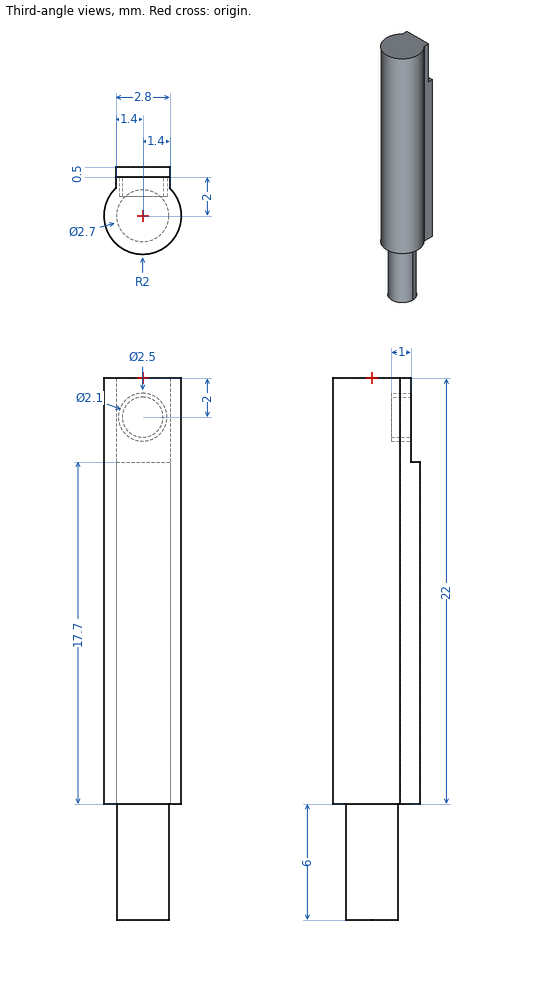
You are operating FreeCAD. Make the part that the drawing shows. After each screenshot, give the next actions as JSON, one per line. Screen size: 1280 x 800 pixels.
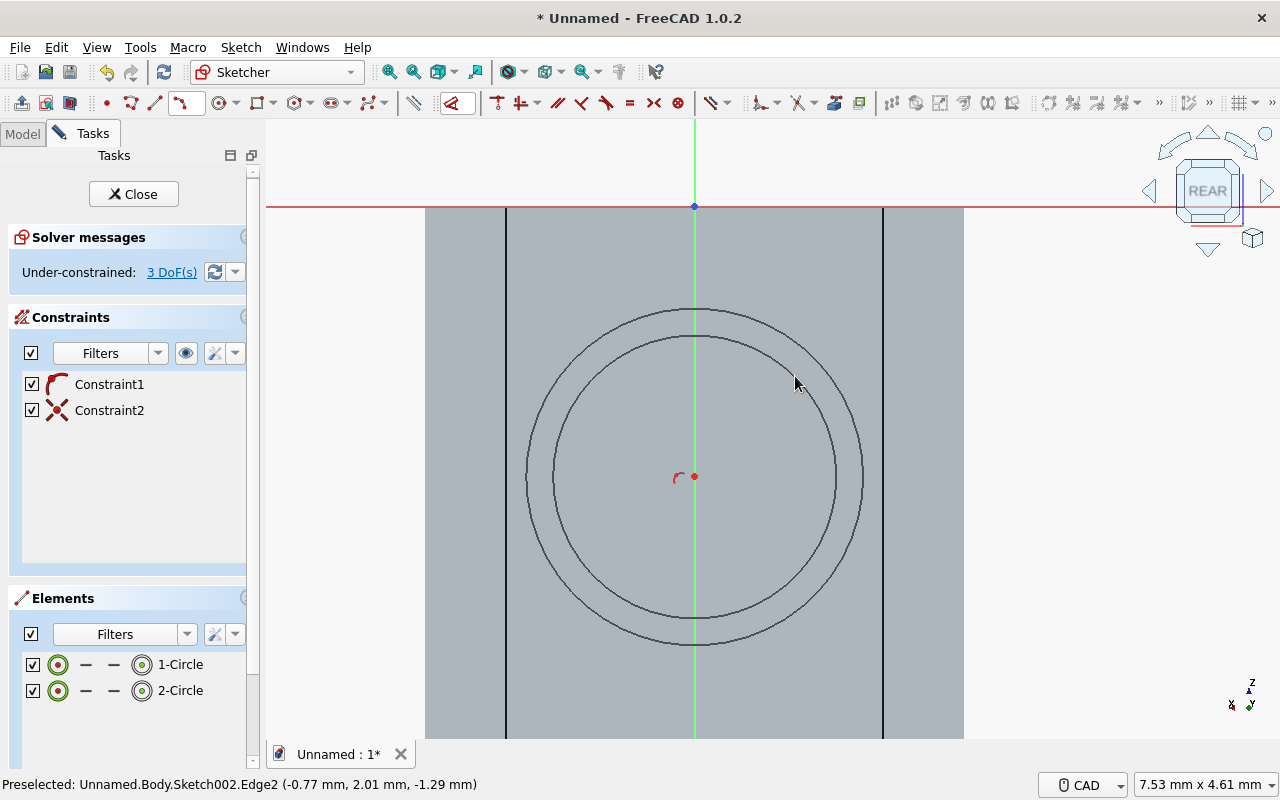
{"action": "left_click", "coordinate": [813, 357]}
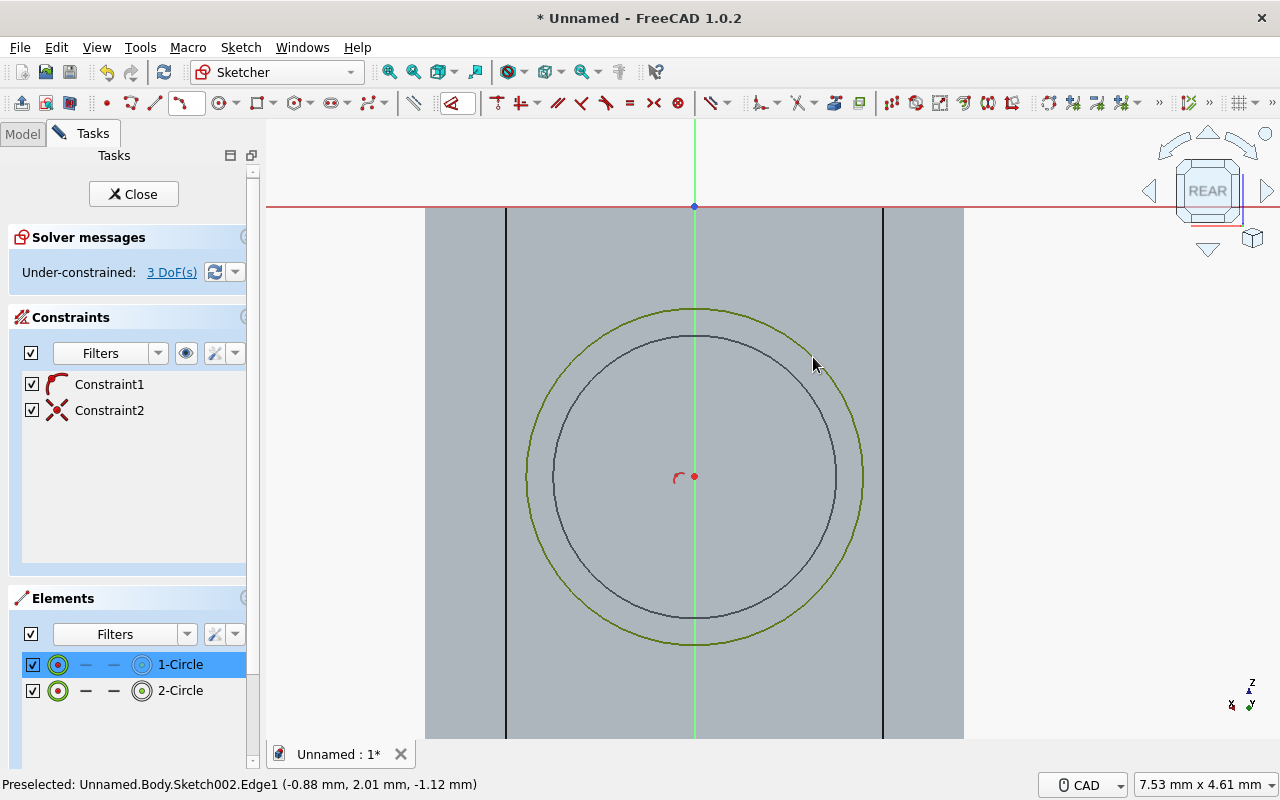
{"action": "key", "text": "k o"}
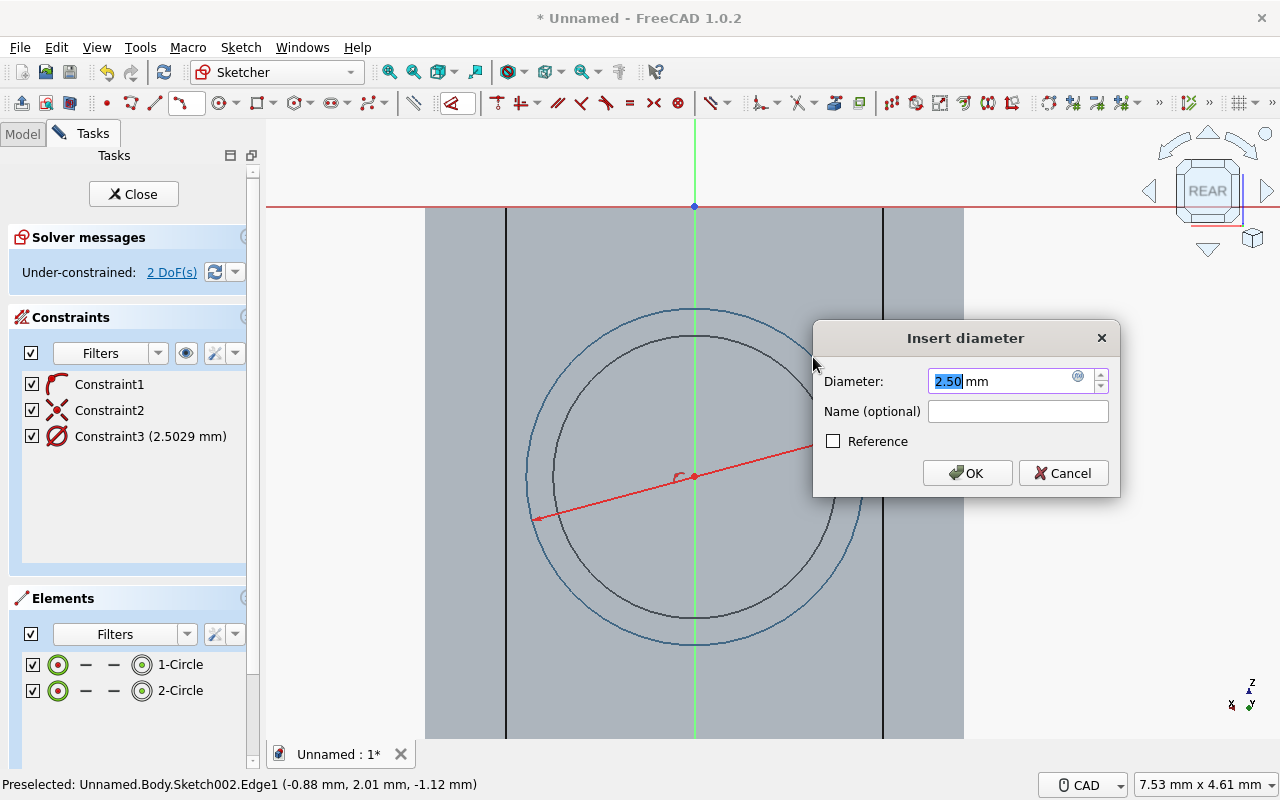
{"action": "type", "text": "2.5"}
{"action": "key", "text": "Return"}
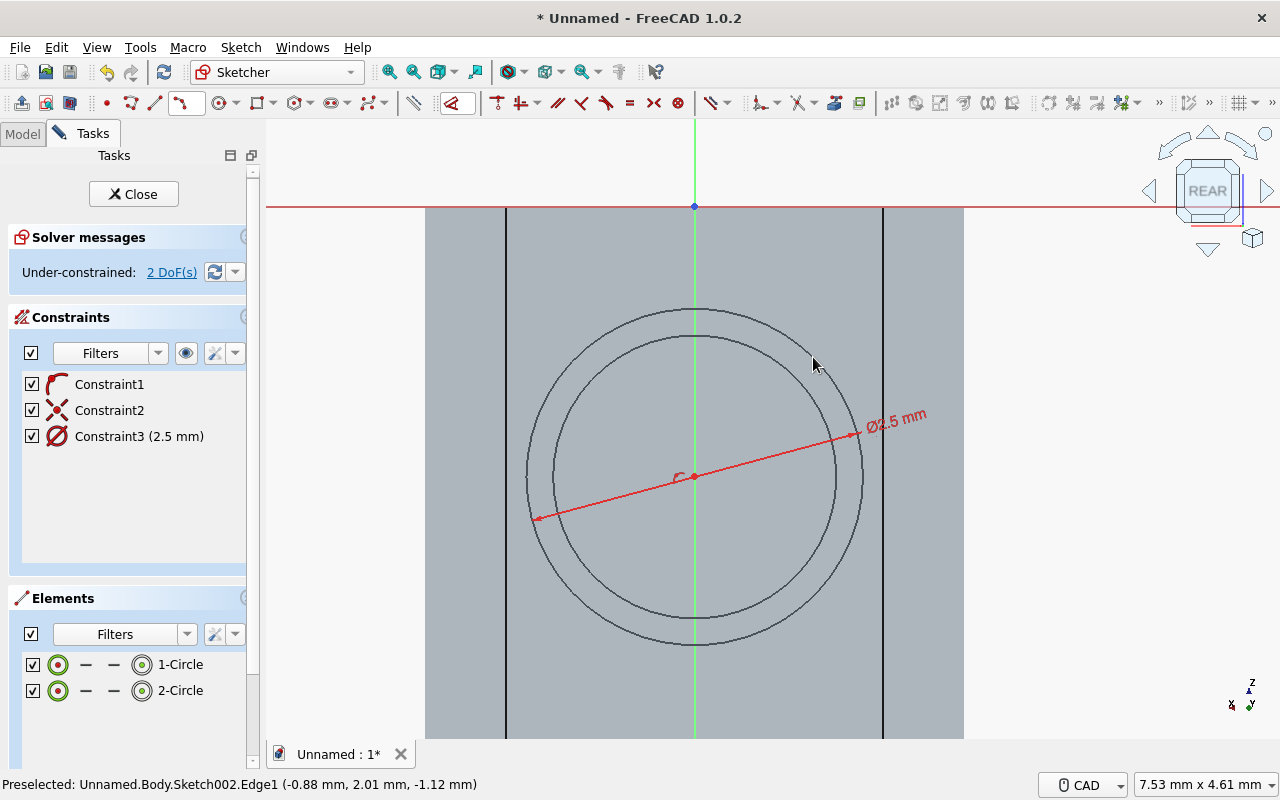
{"action": "left_click", "coordinate": [795, 377]}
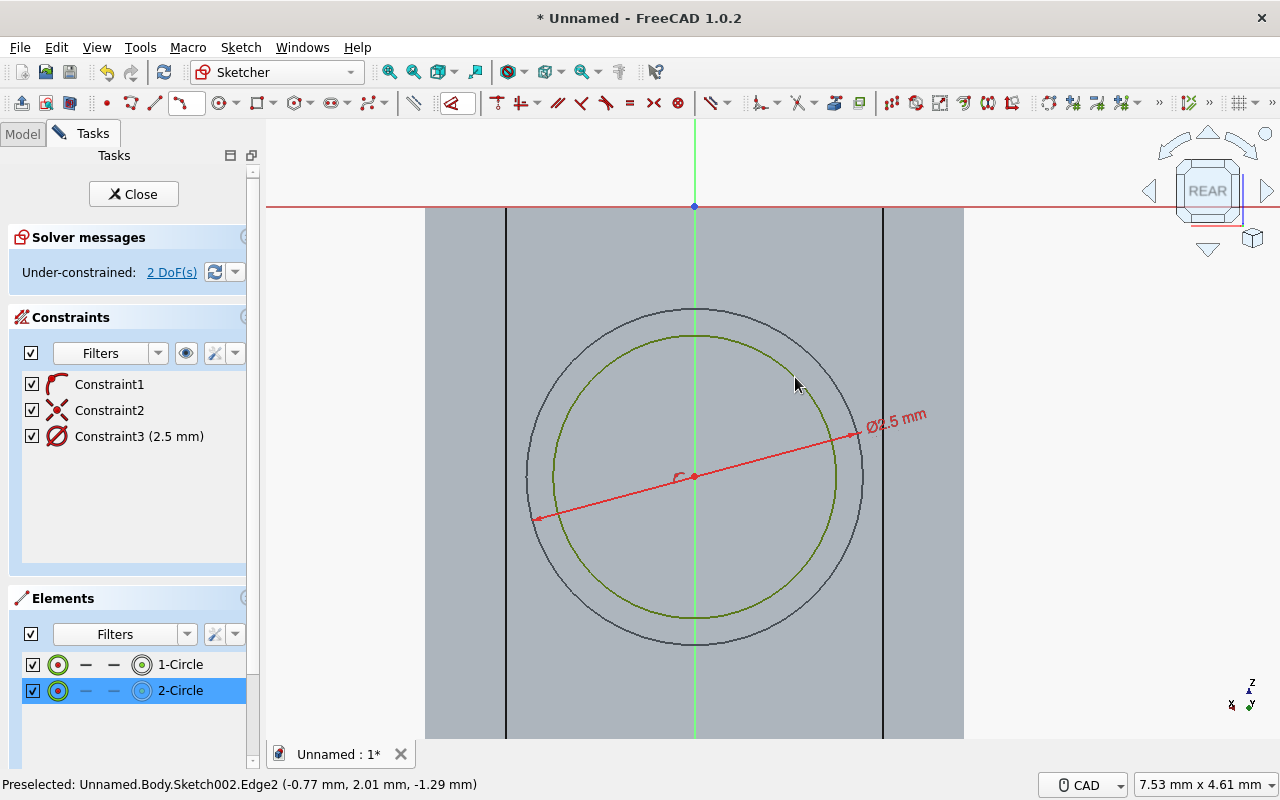
{"action": "left_click", "coordinate": [470, 104]}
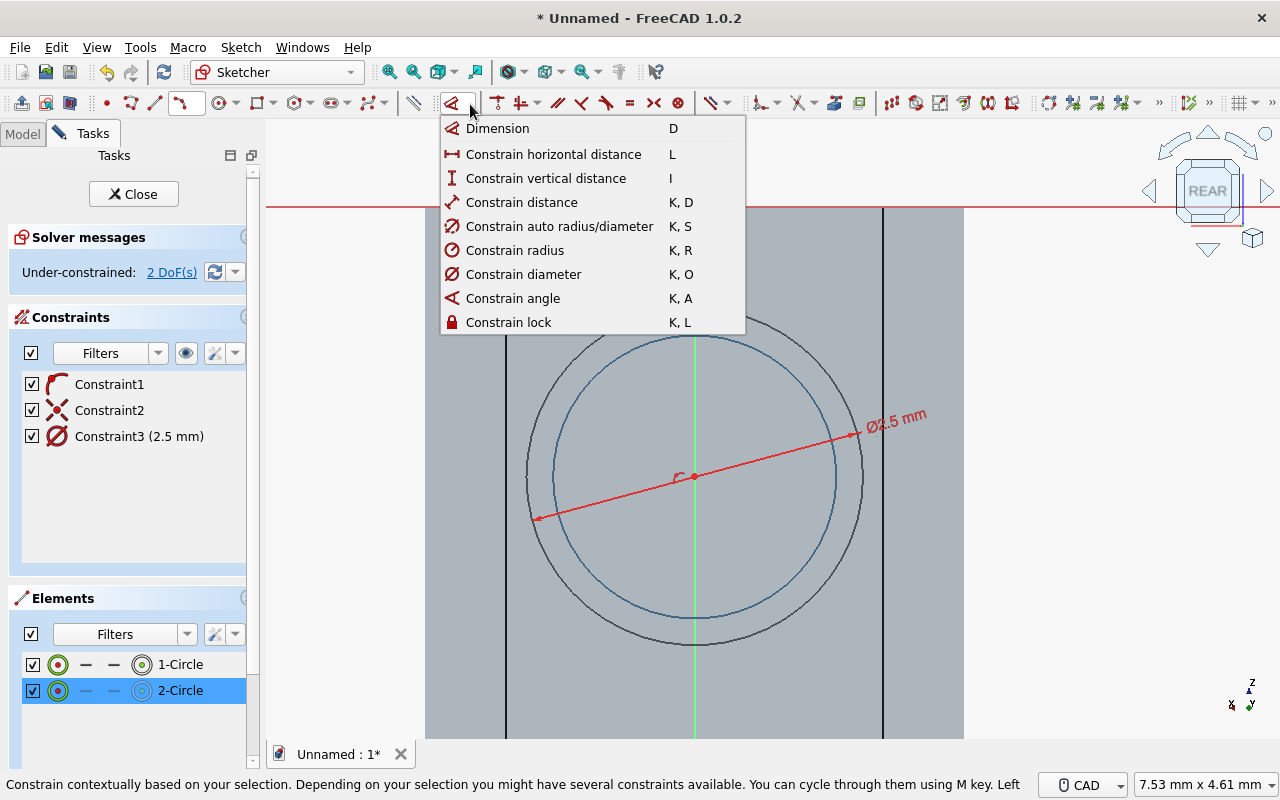
{"action": "left_click", "coordinate": [593, 274]}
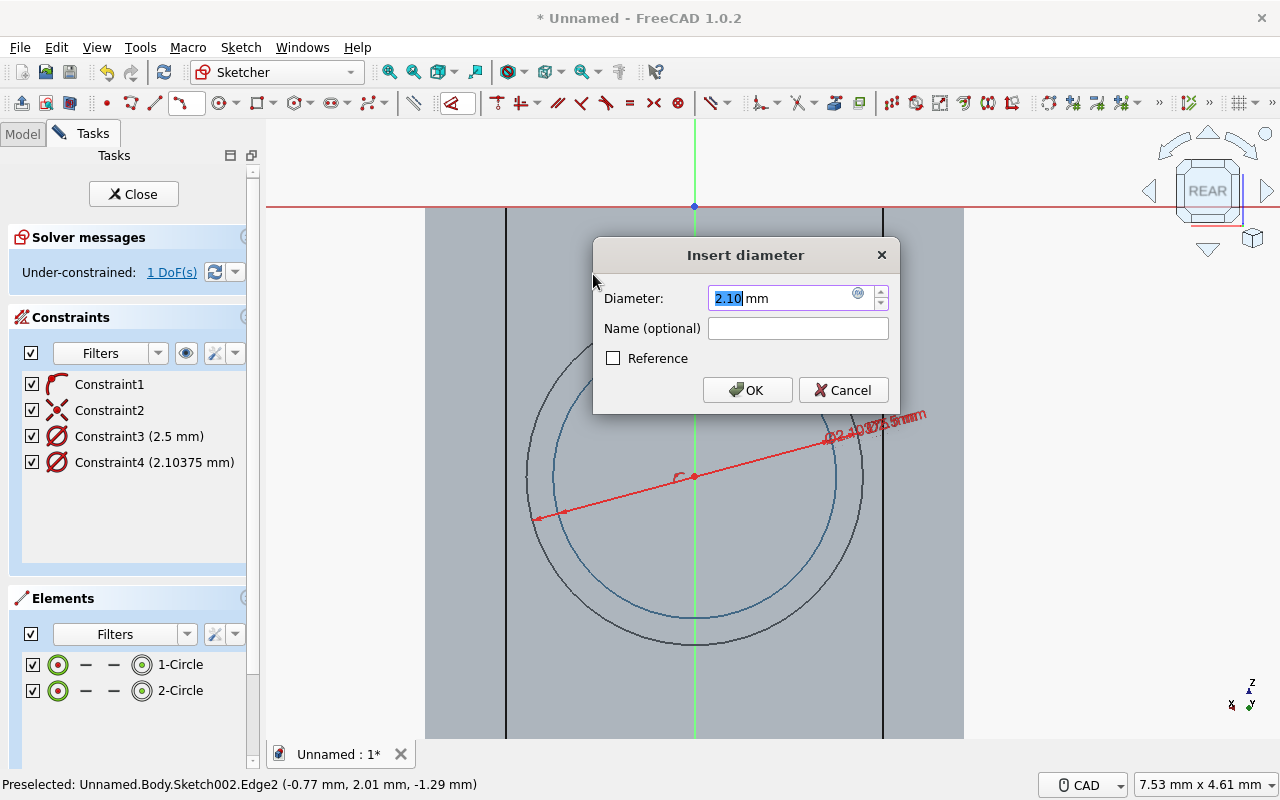
{"action": "type", "text": "2.1"}
{"action": "key", "text": "Return"}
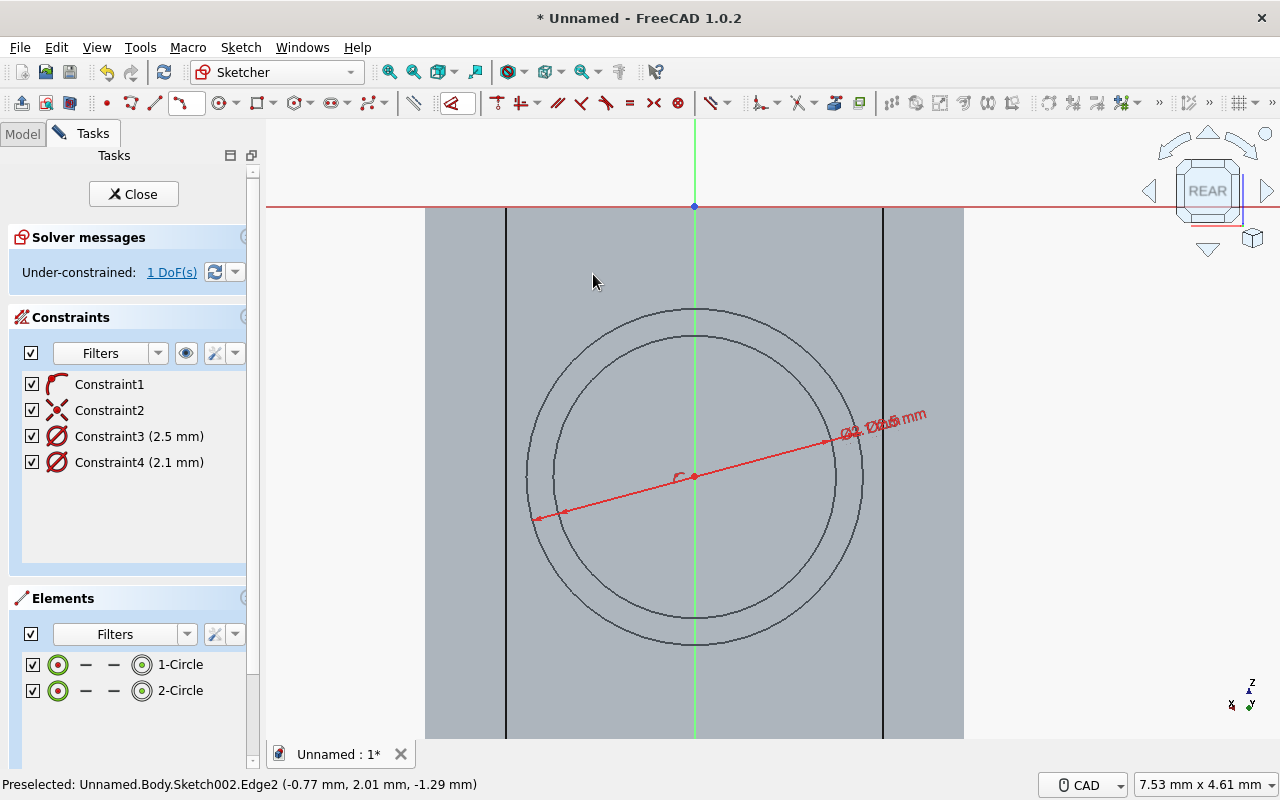
{"action": "left_click", "coordinate": [695, 477]}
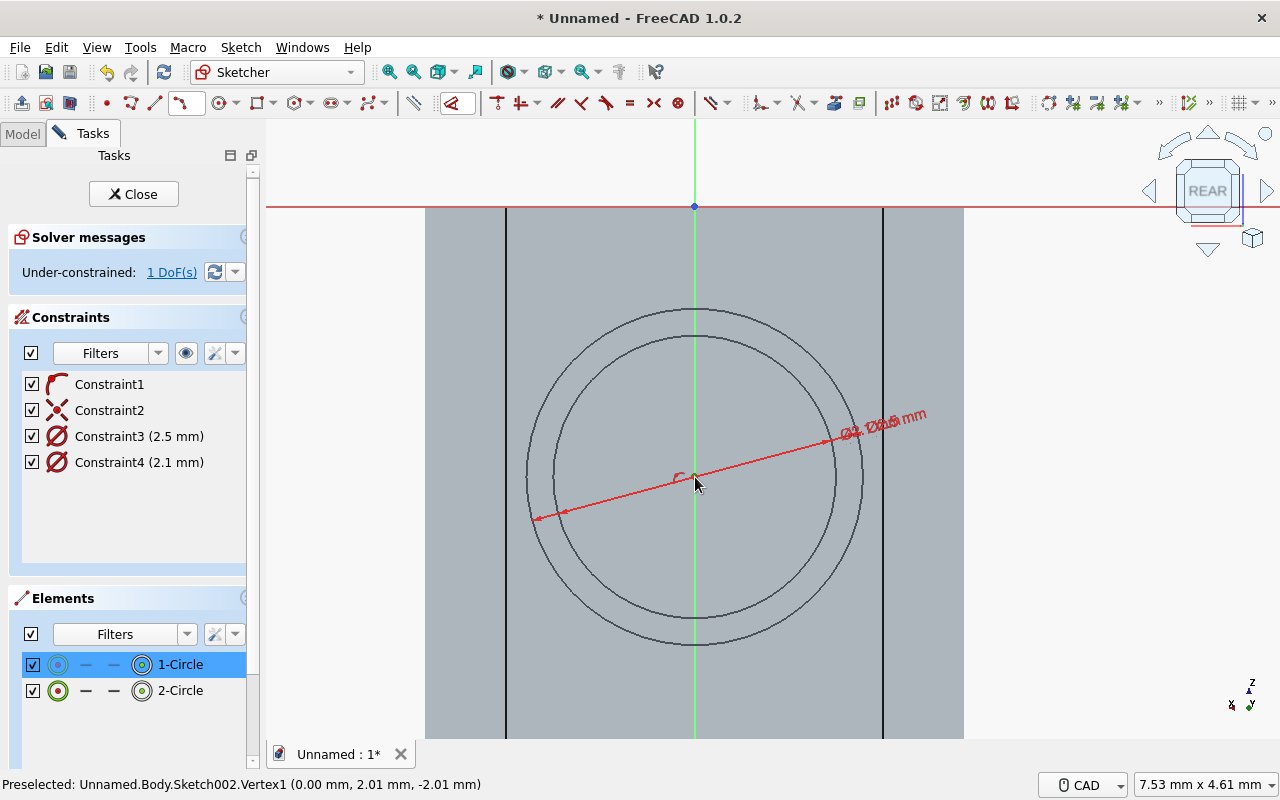
{"action": "left_click", "coordinate": [470, 104]}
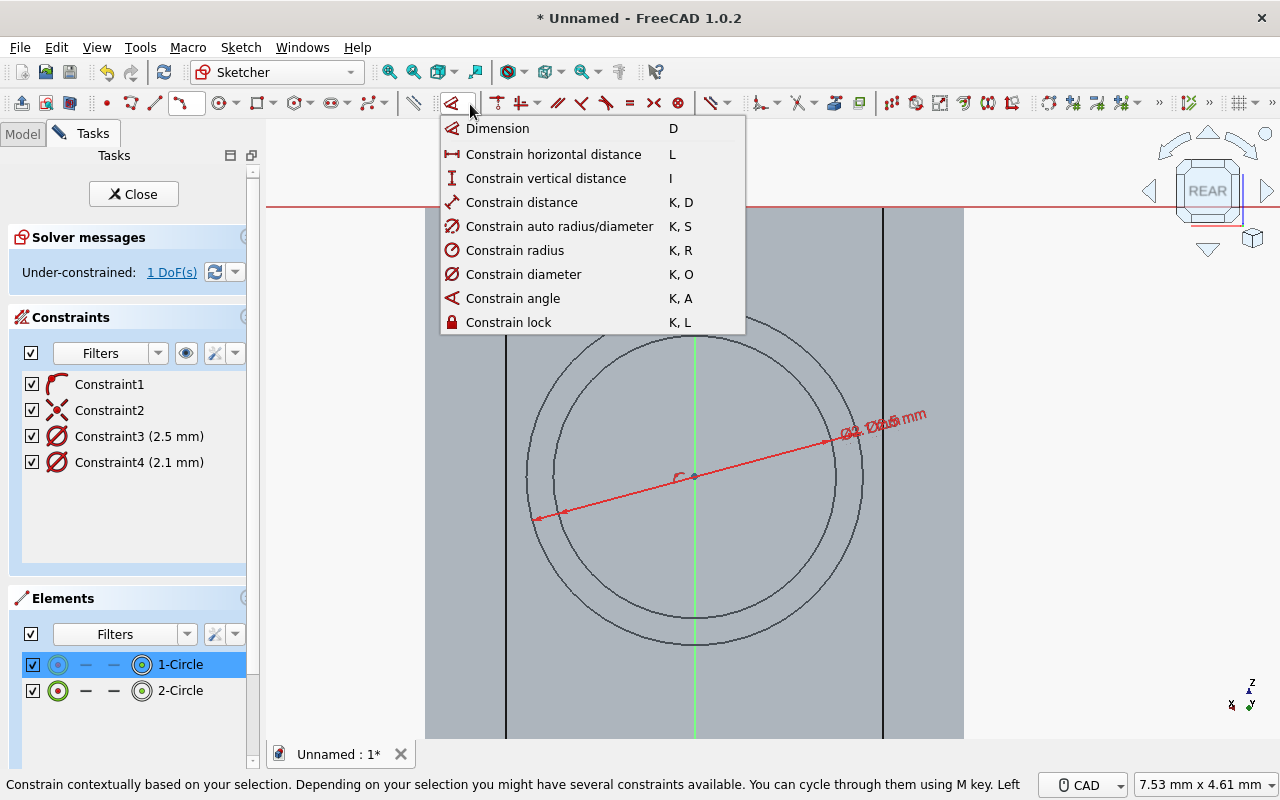
{"action": "left_click", "coordinate": [593, 178]}